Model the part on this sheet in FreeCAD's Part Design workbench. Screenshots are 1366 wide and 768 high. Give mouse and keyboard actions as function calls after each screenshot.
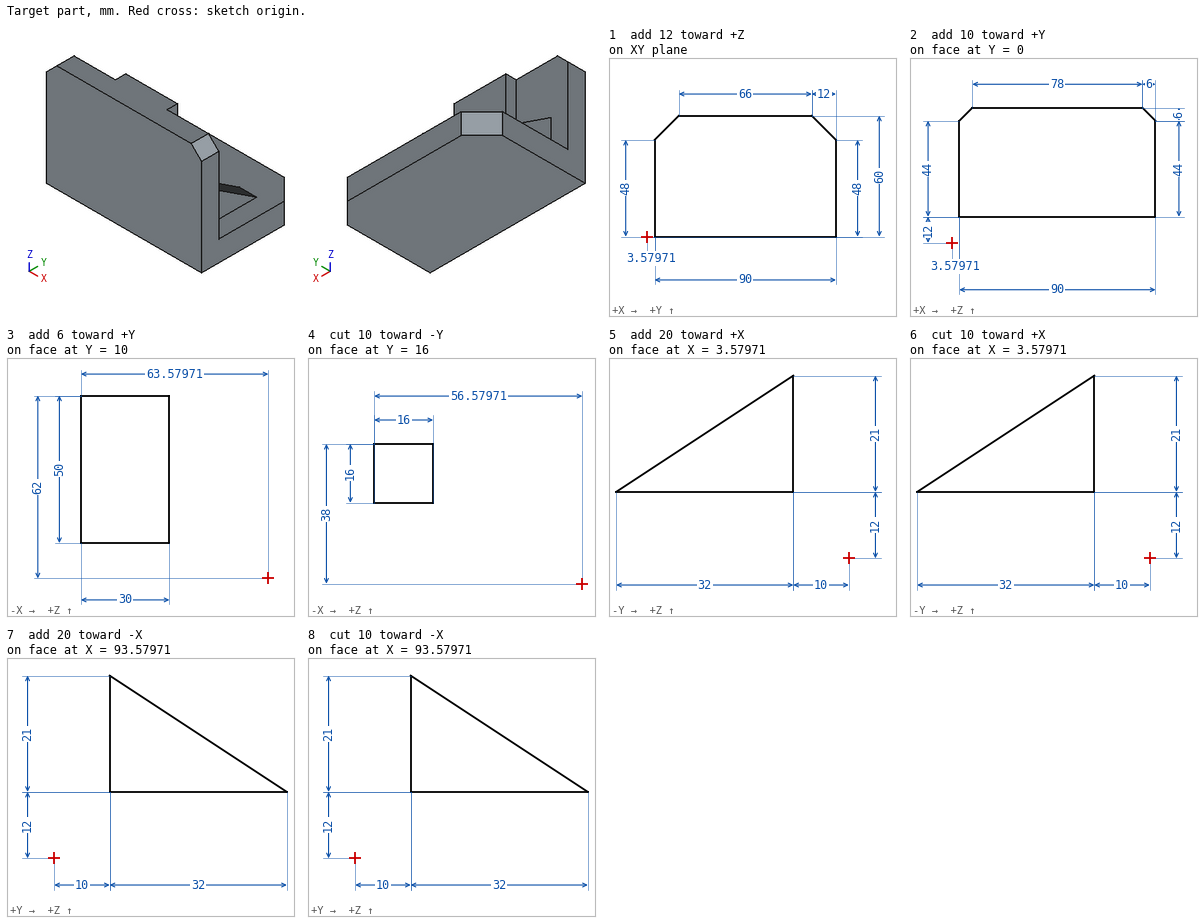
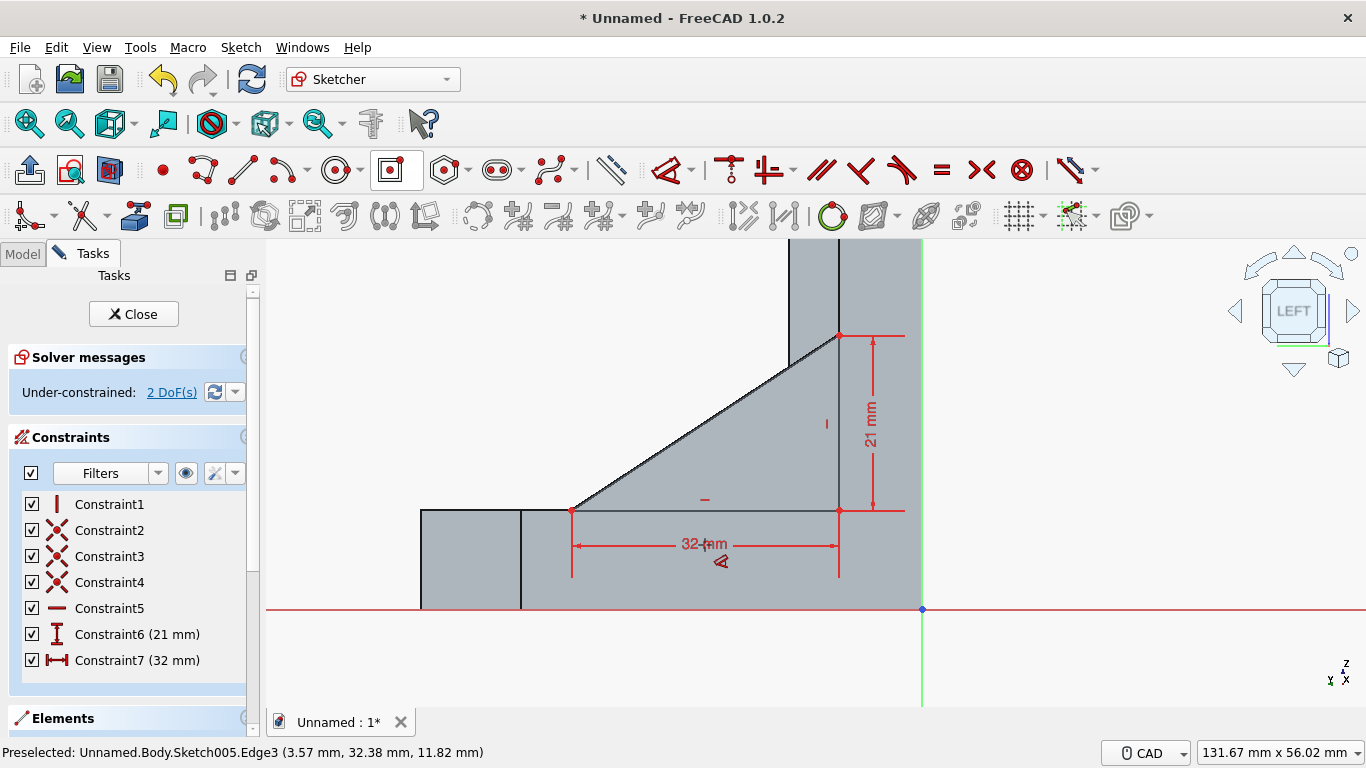
click(839, 511)
click(881, 644)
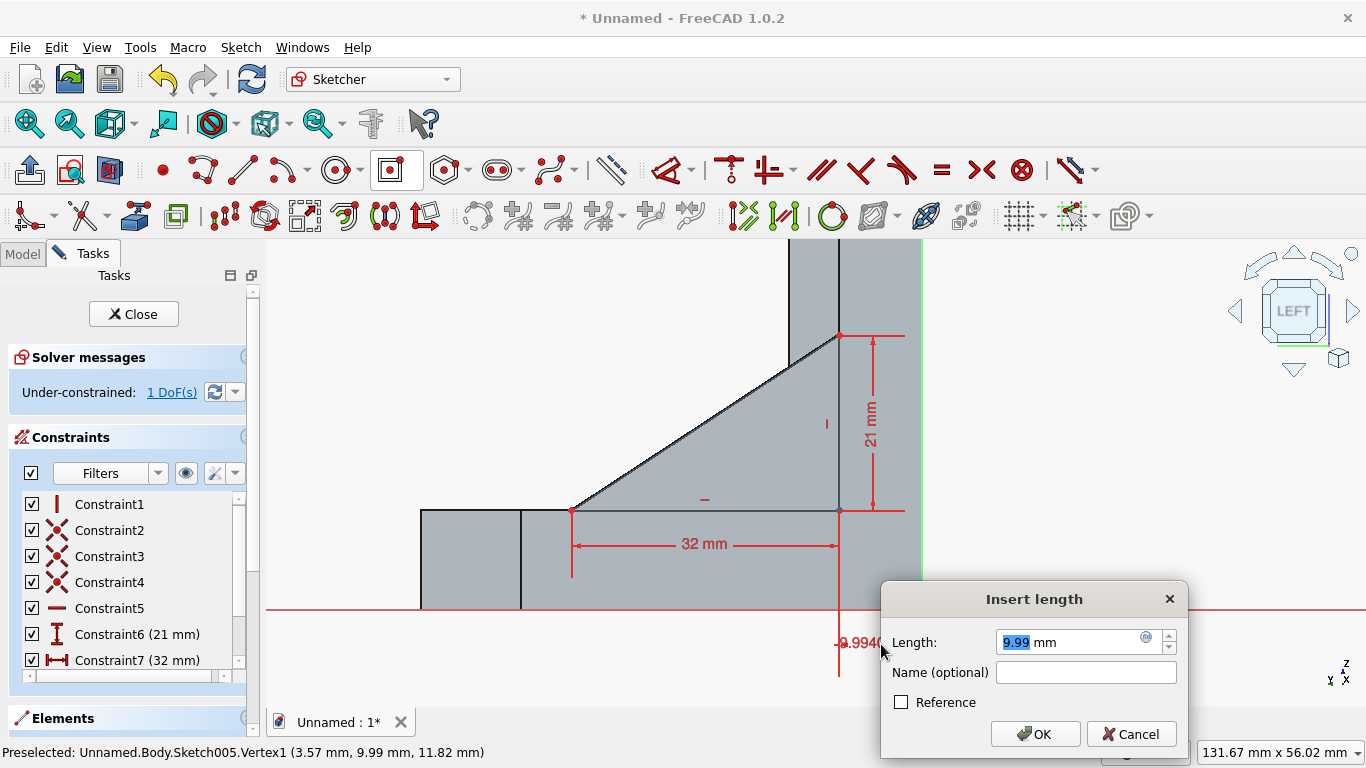
text(10)
key(Return)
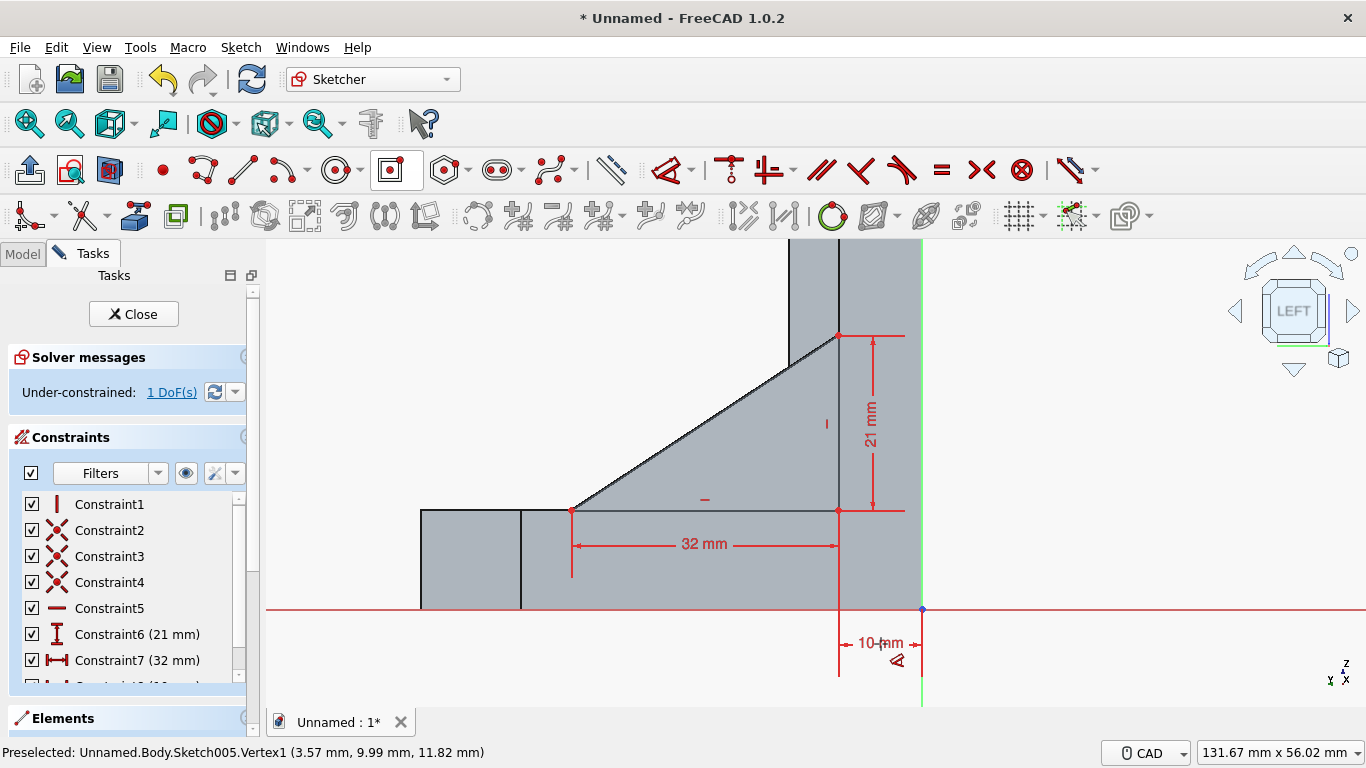
click(839, 511)
click(956, 560)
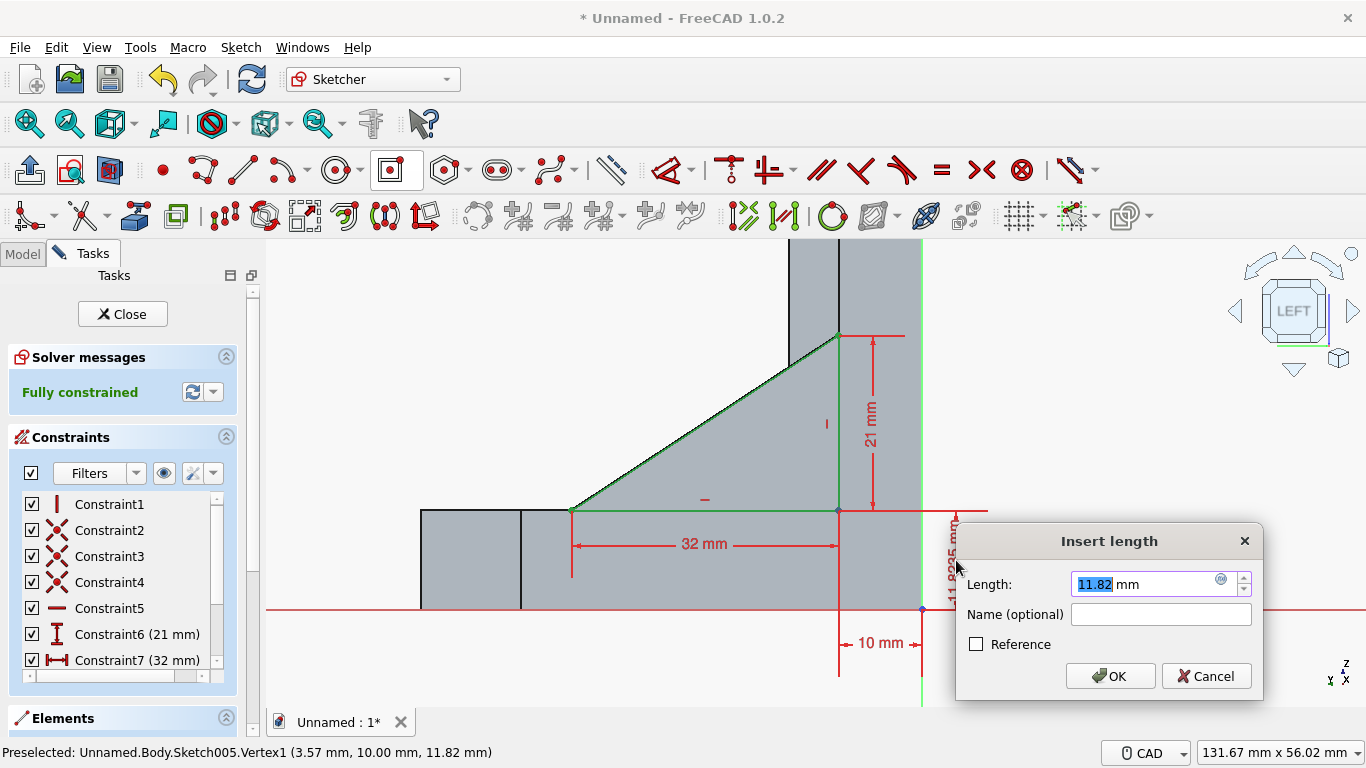
text(12)
key(Return)
key(Escape)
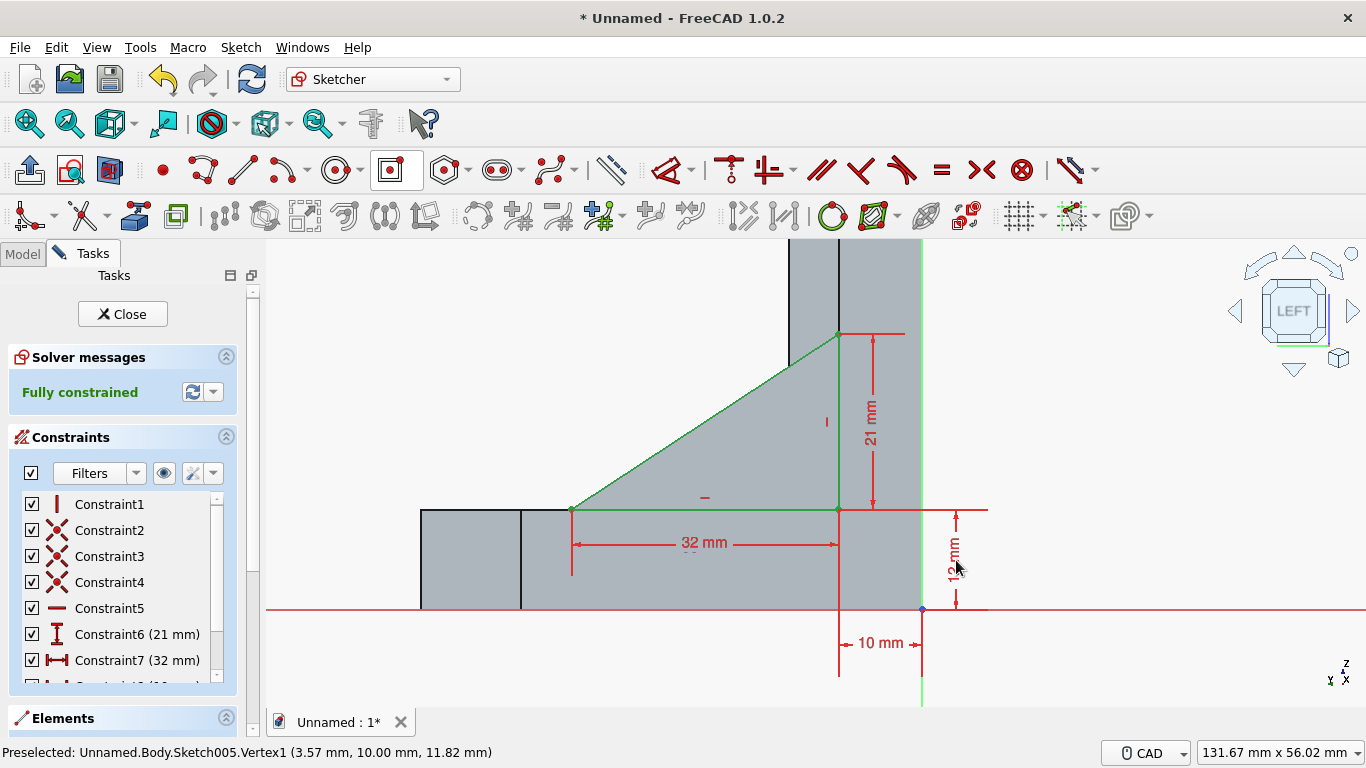
click(123, 314)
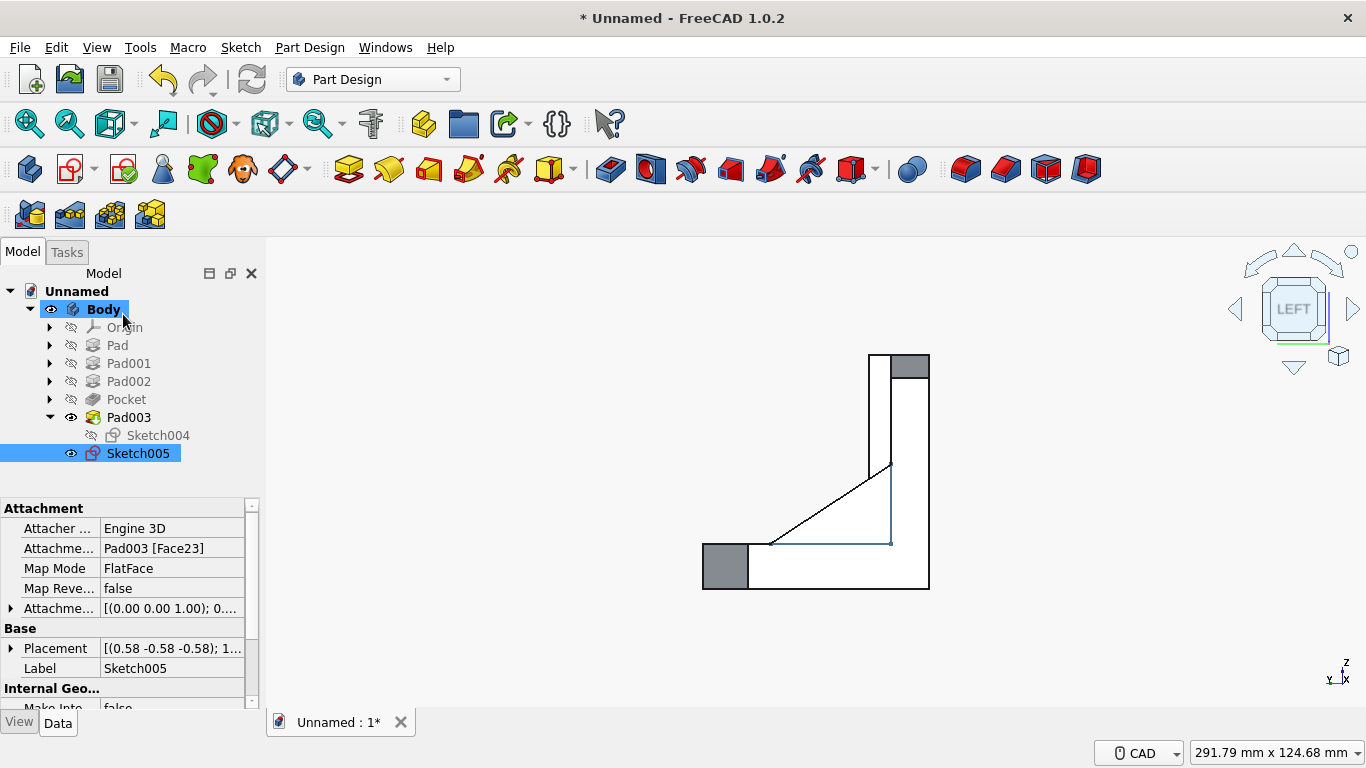
click(612, 170)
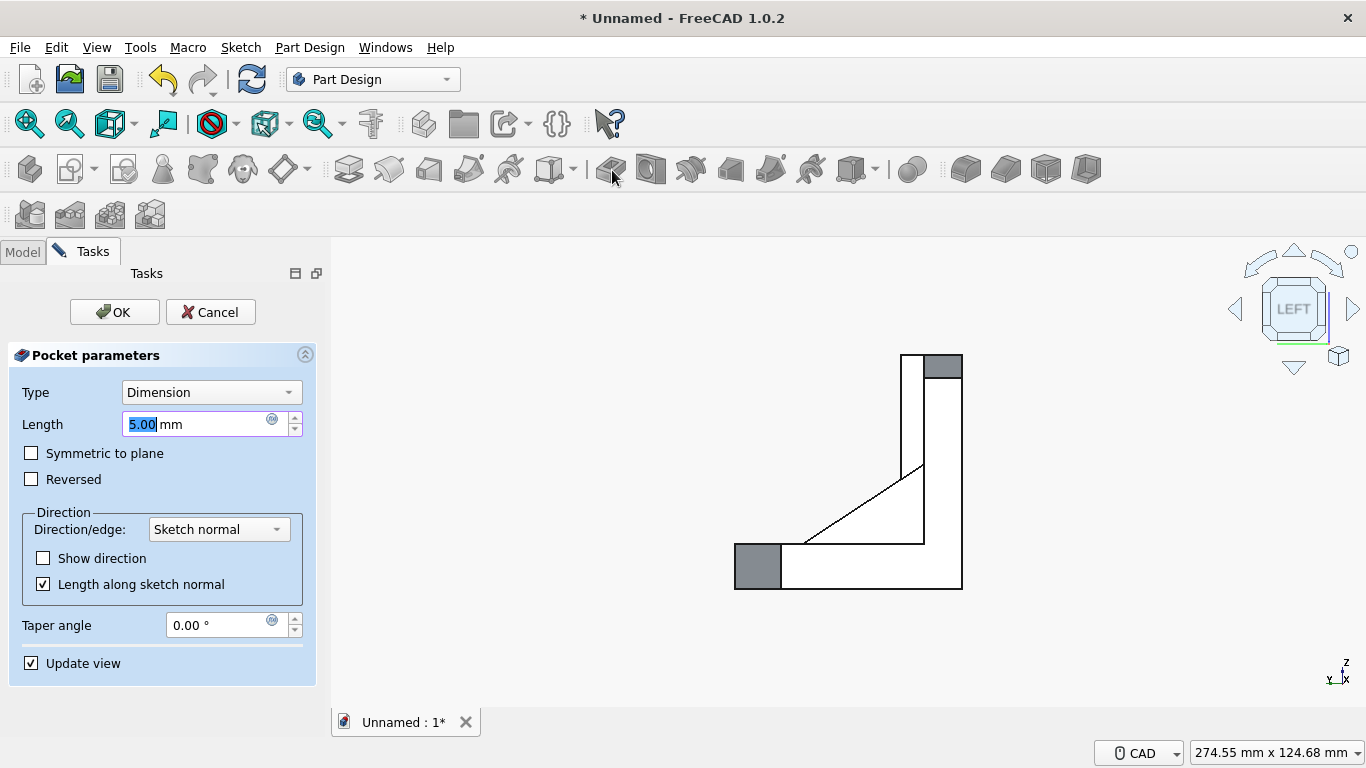
text(10)
key(Tab)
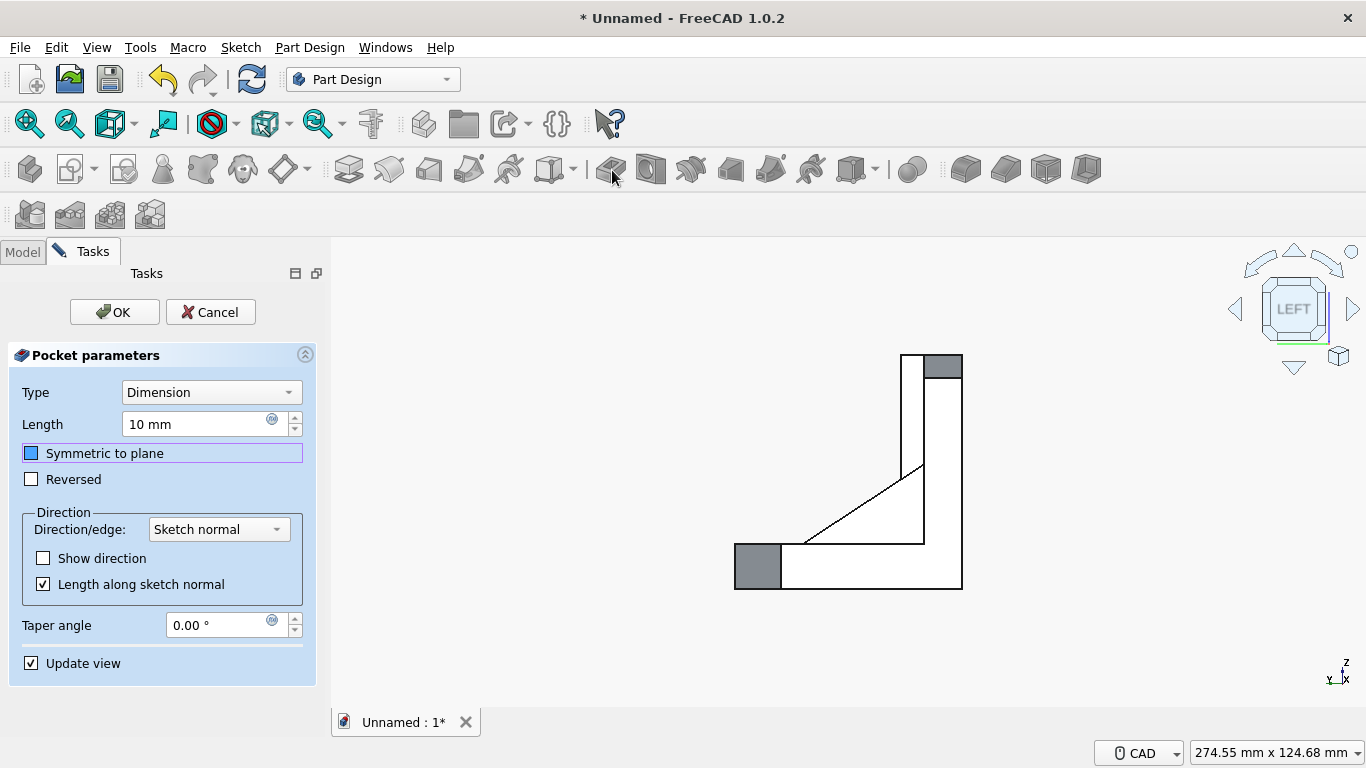
click(115, 312)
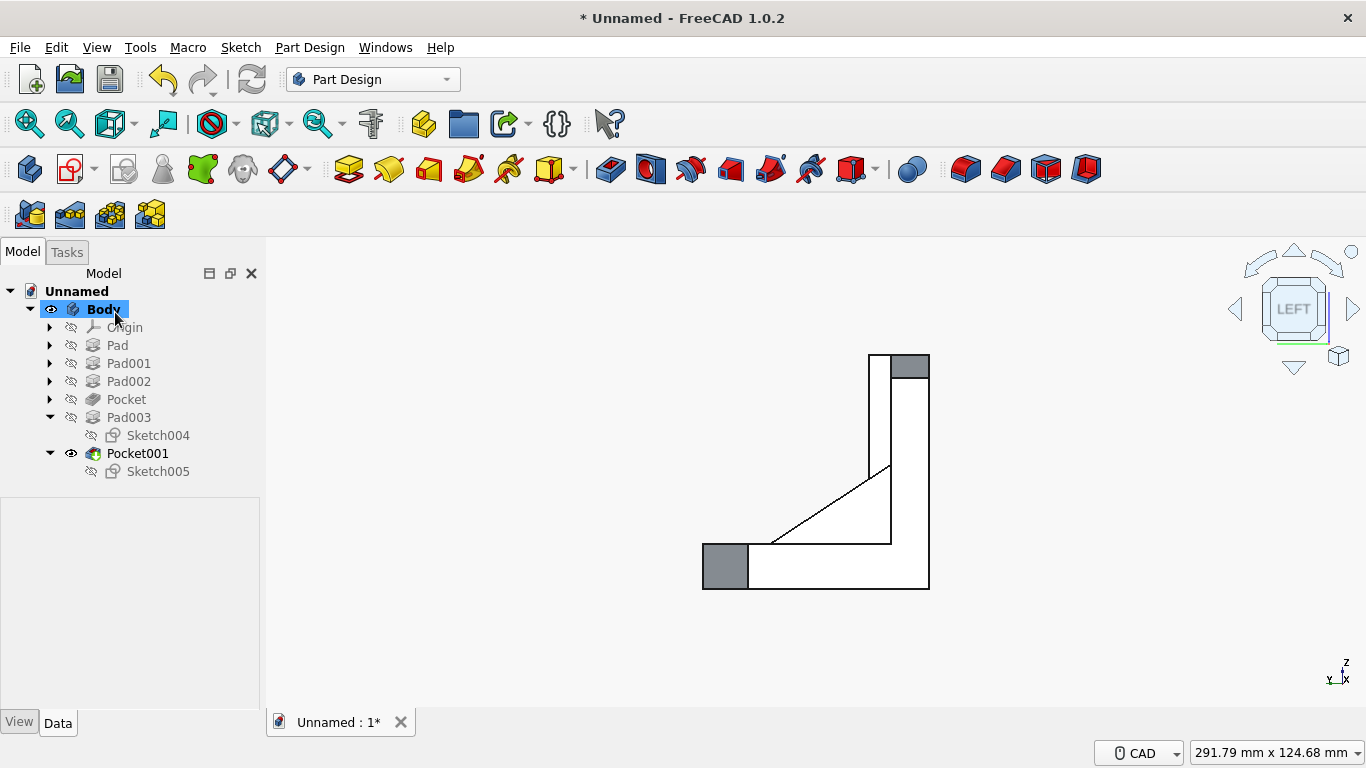
key(0)